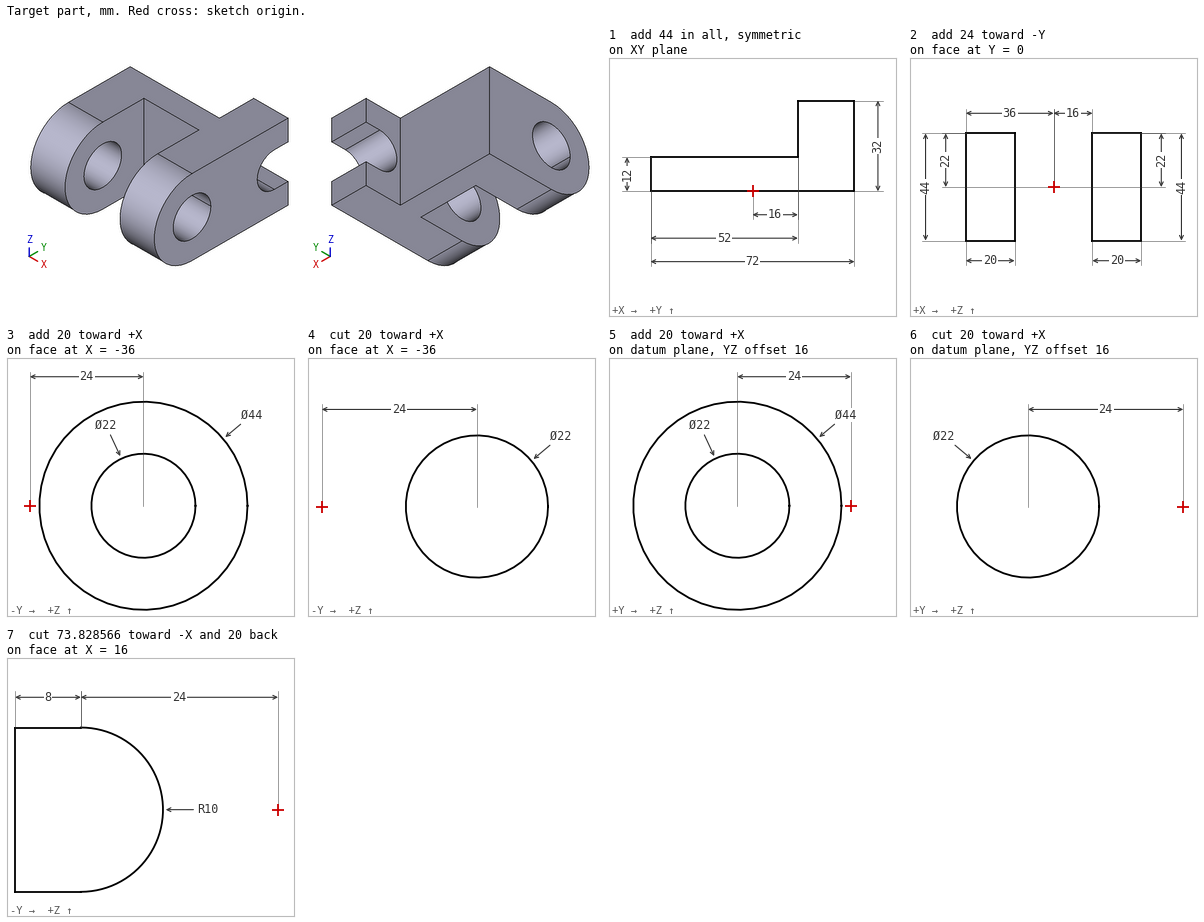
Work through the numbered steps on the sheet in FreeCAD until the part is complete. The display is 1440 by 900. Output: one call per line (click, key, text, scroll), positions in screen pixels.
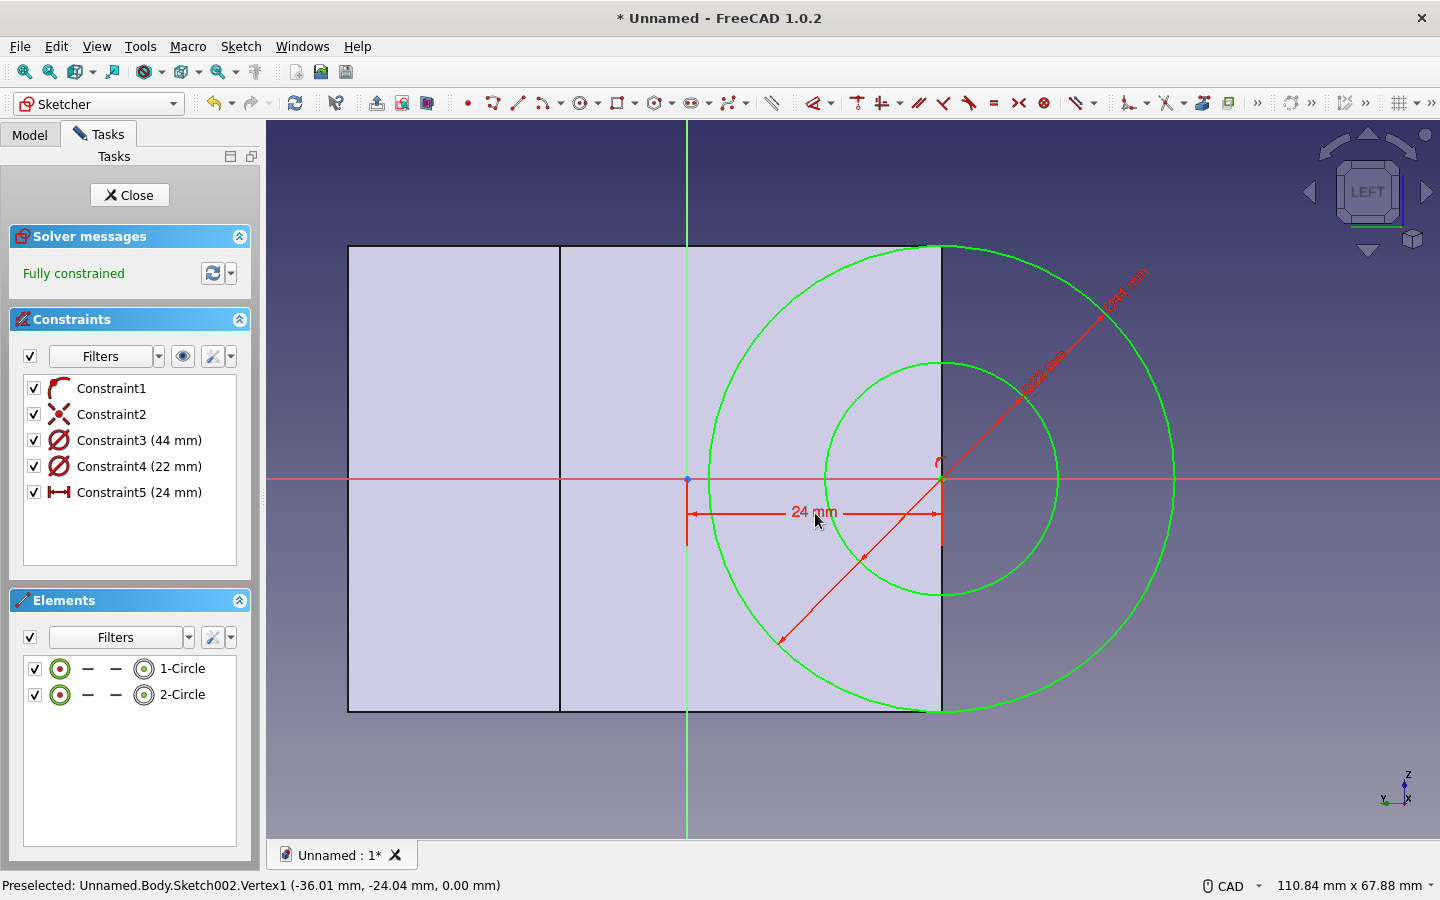
click(130, 195)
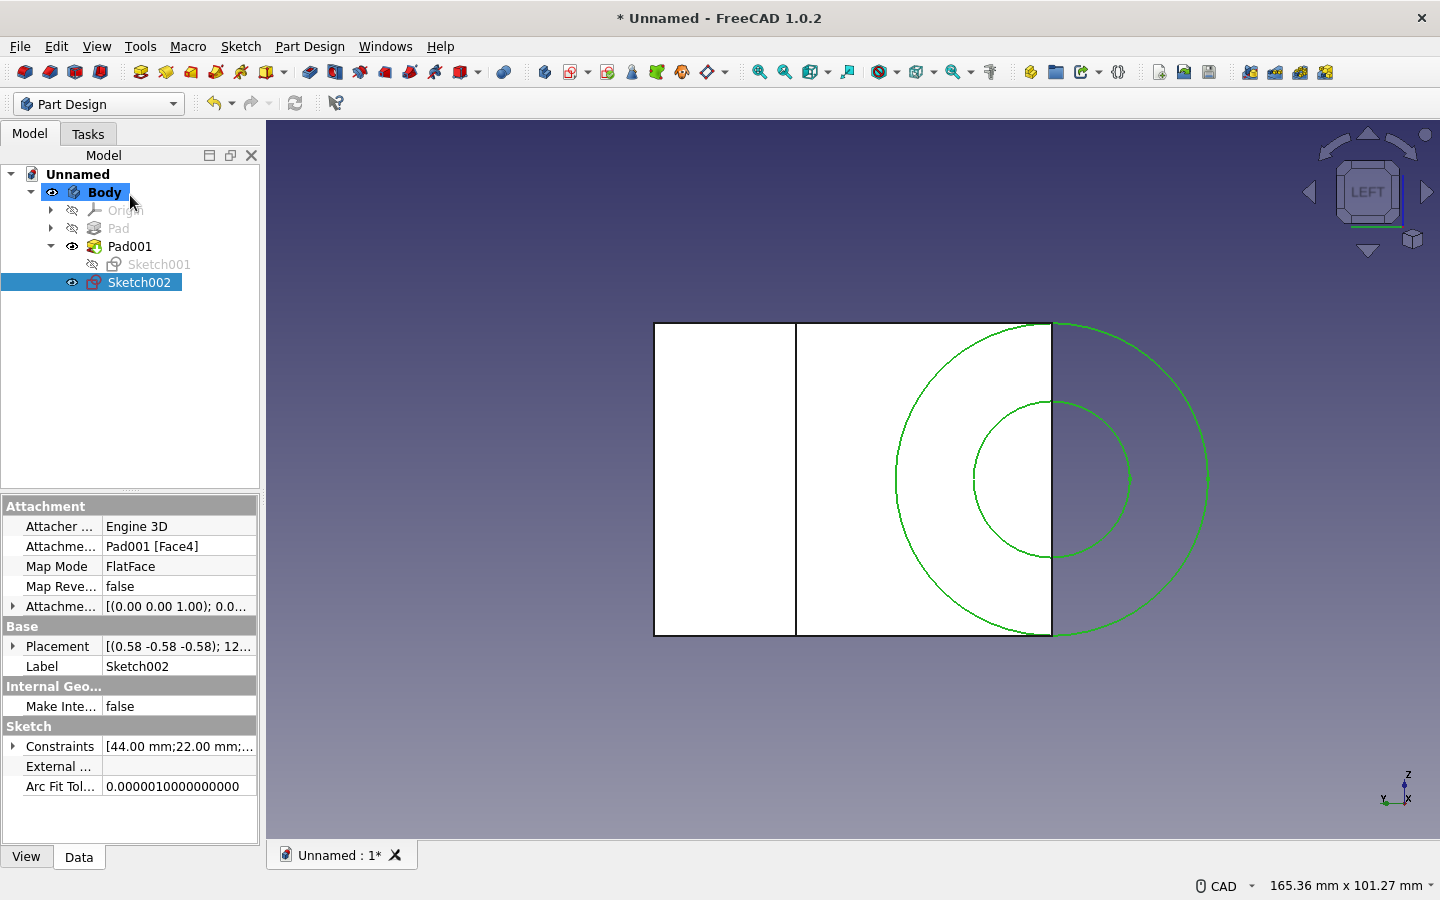
click(141, 72)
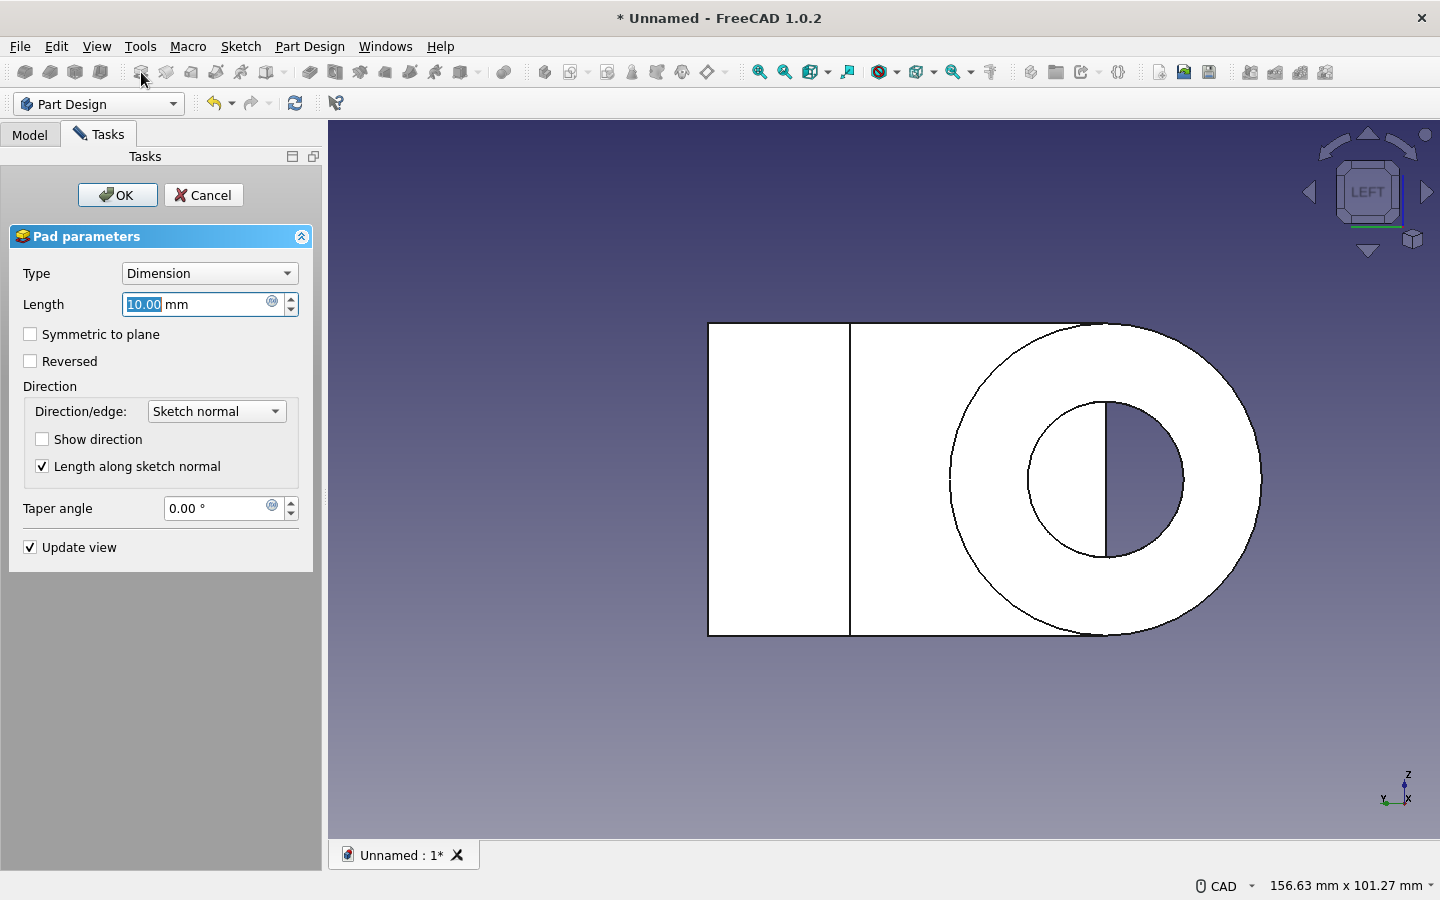
text(20)
key(Tab)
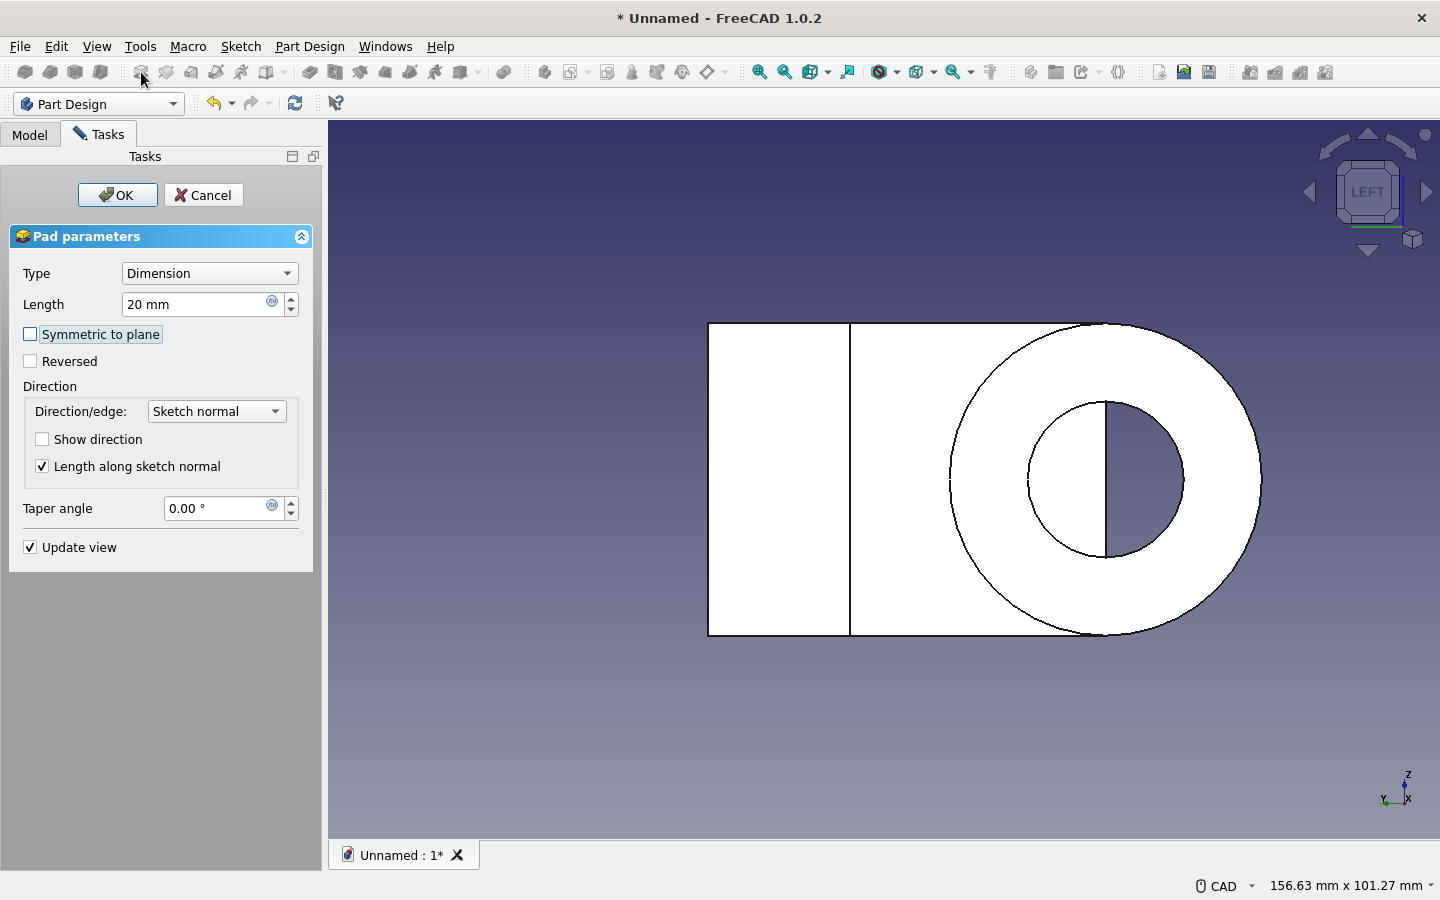
click(31, 361)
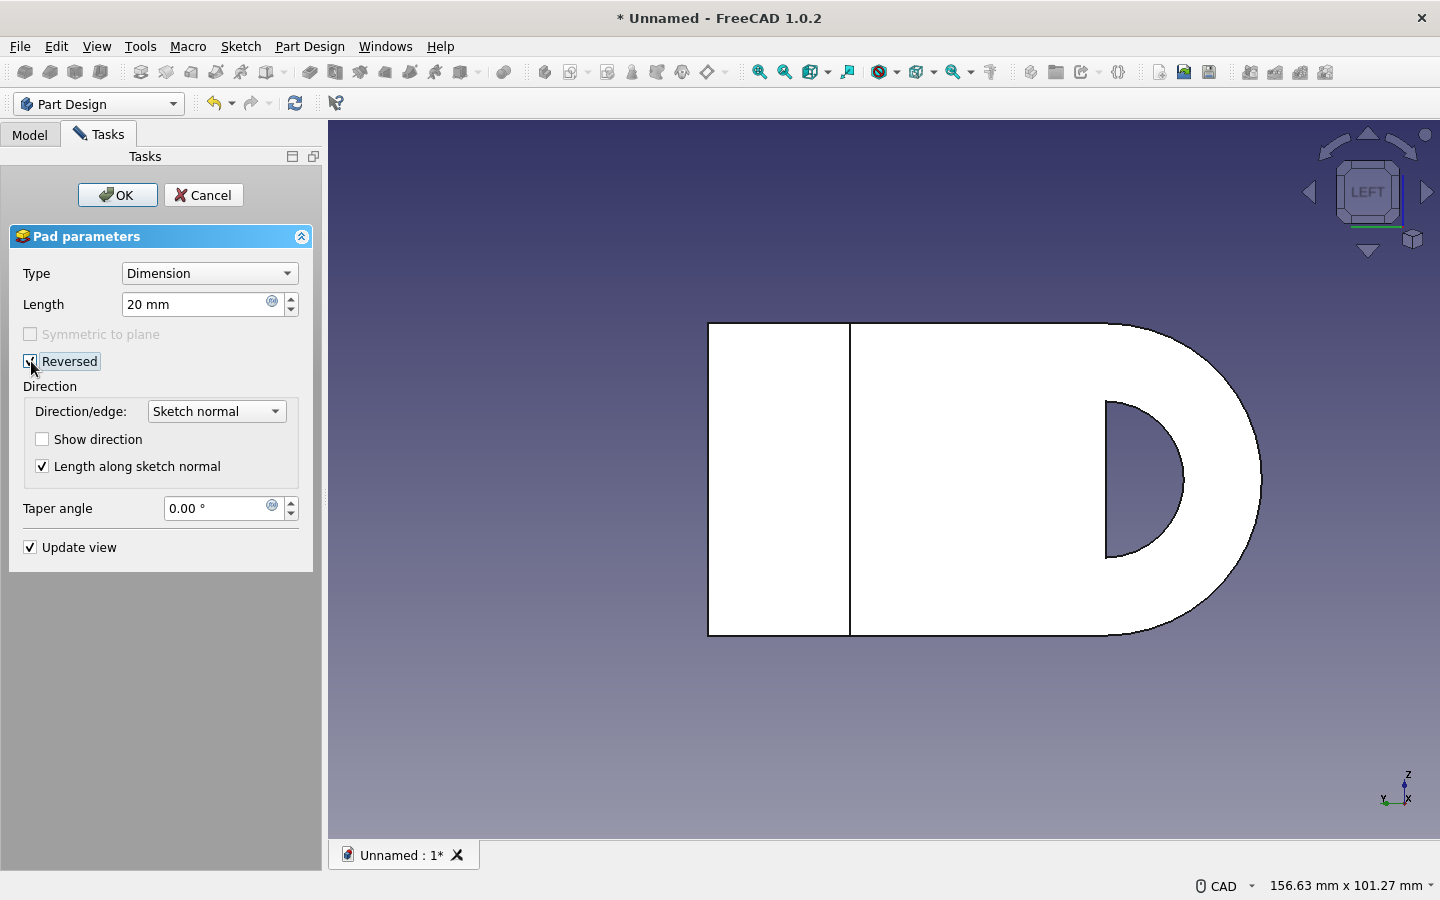
click(118, 195)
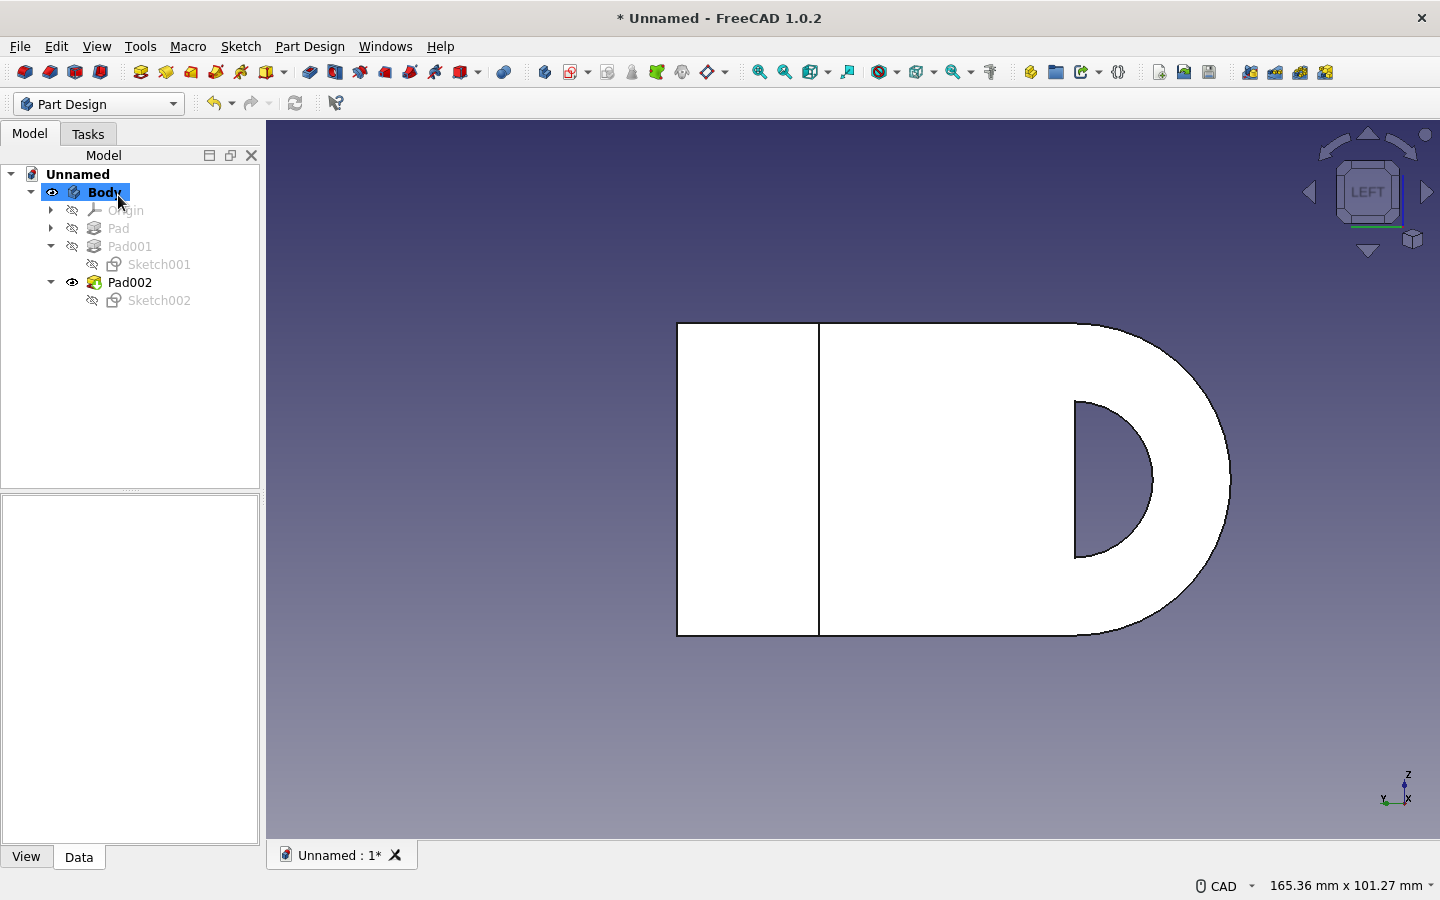
click(966, 523)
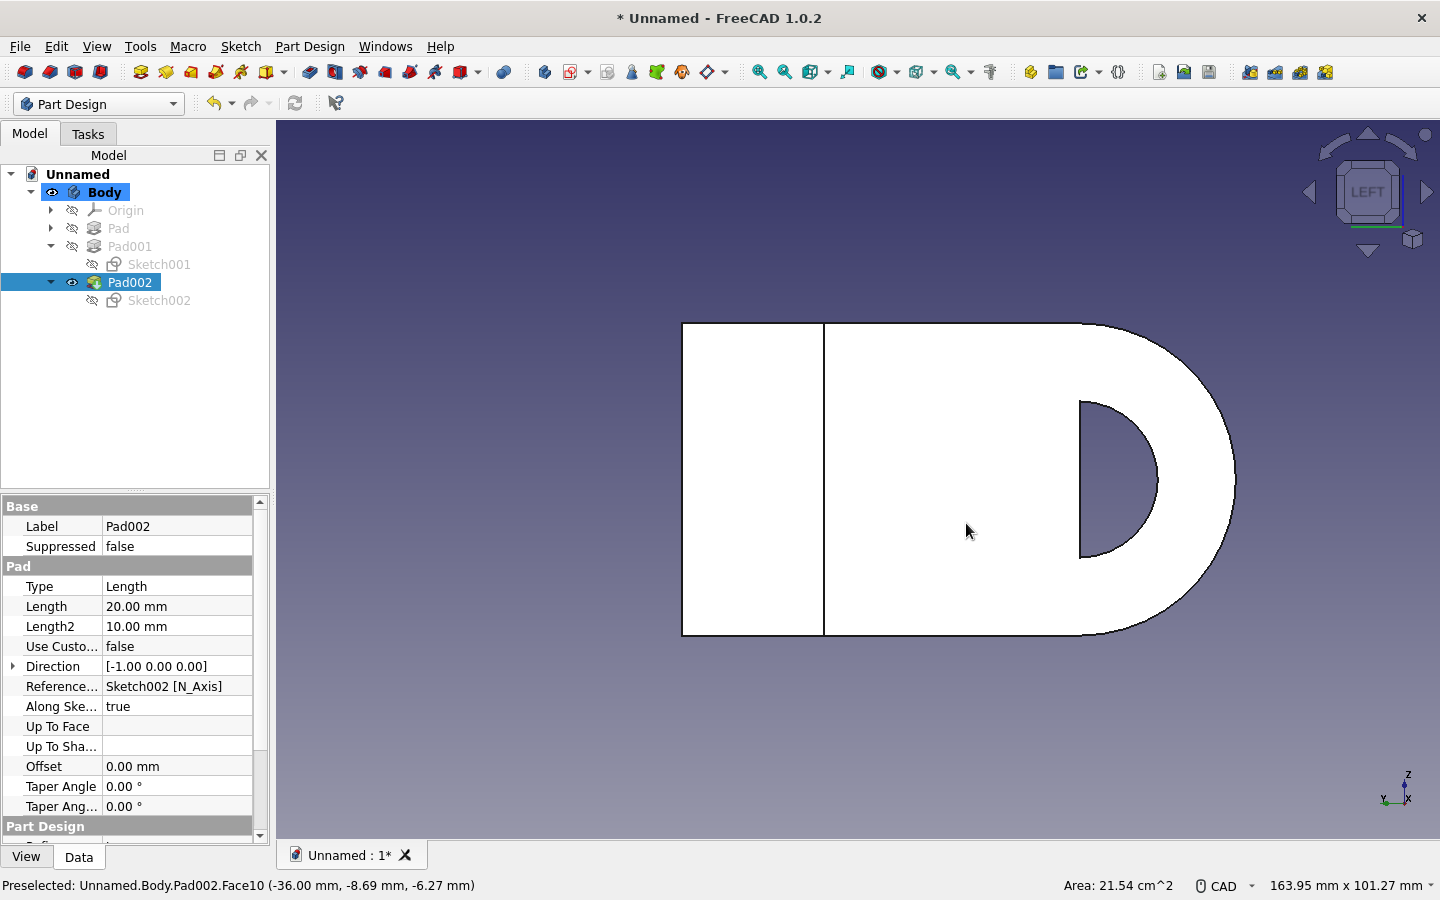
click(570, 72)